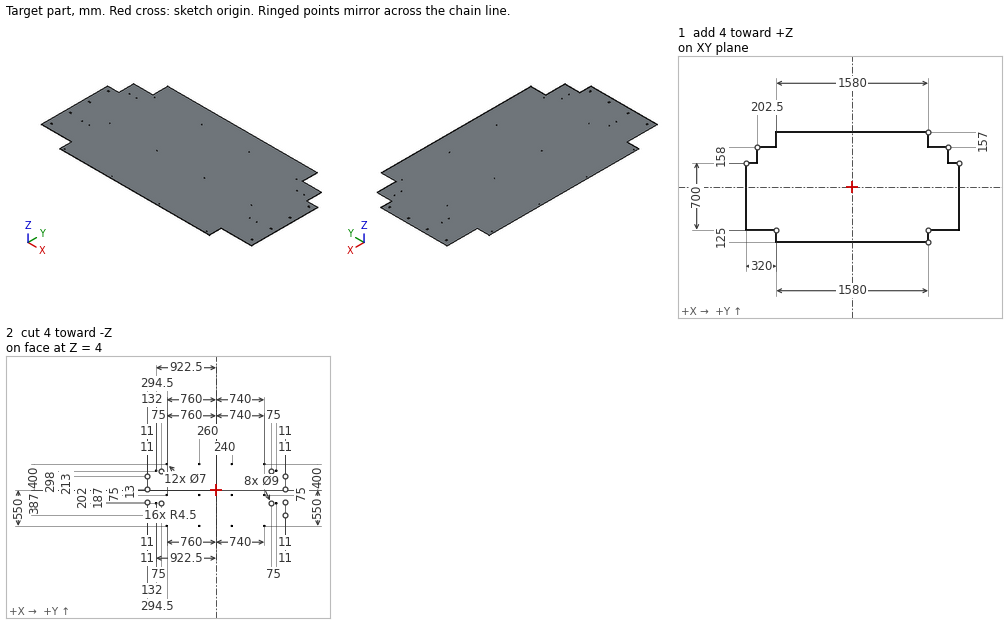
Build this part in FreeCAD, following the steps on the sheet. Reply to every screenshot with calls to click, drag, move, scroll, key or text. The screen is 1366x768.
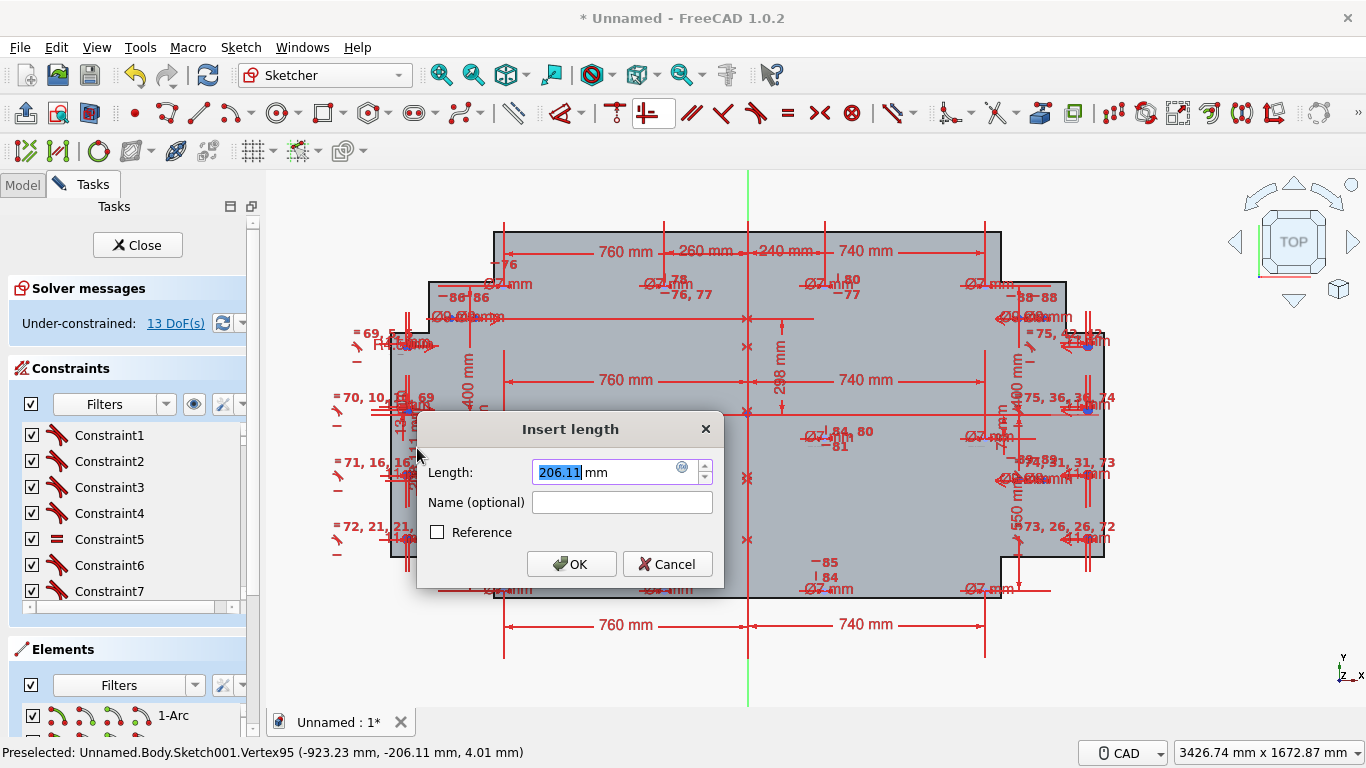
text(202)
key(Return)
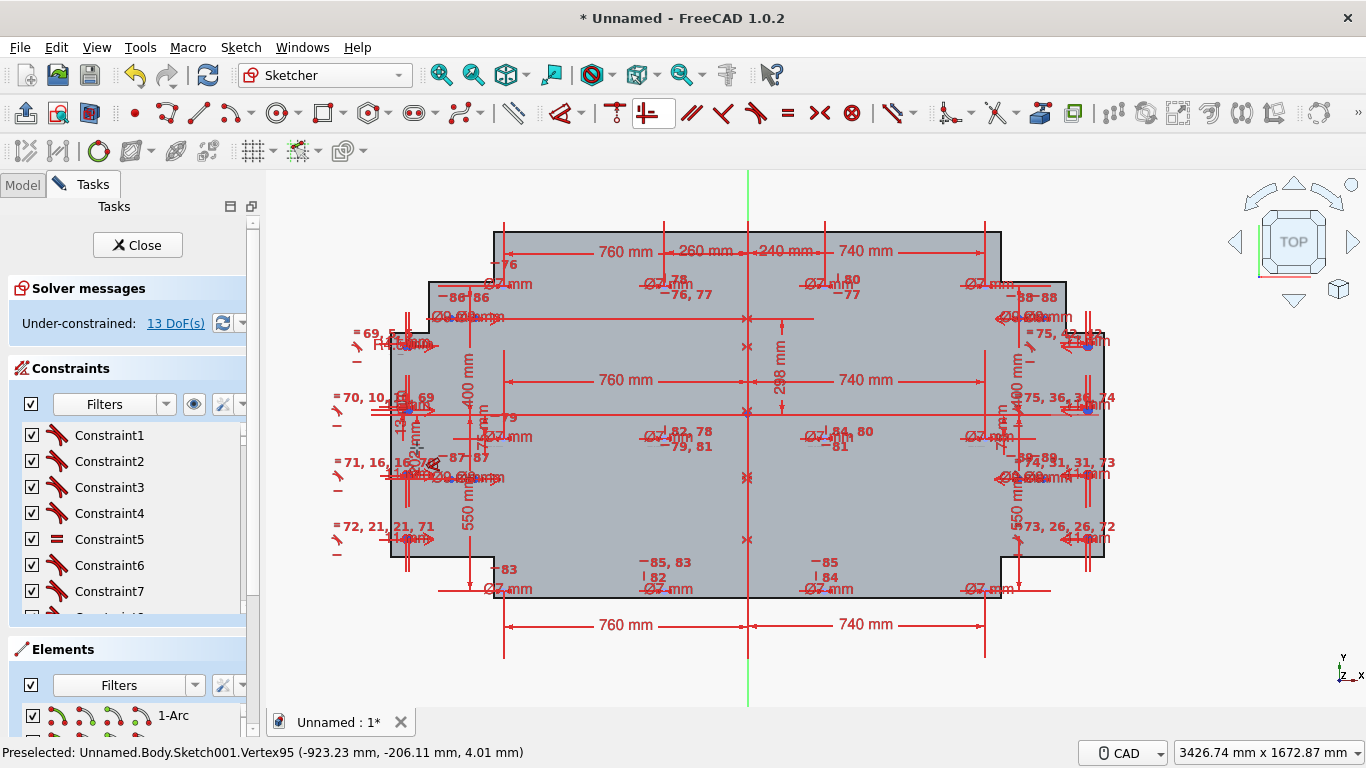
scroll(451, 319, up, 3)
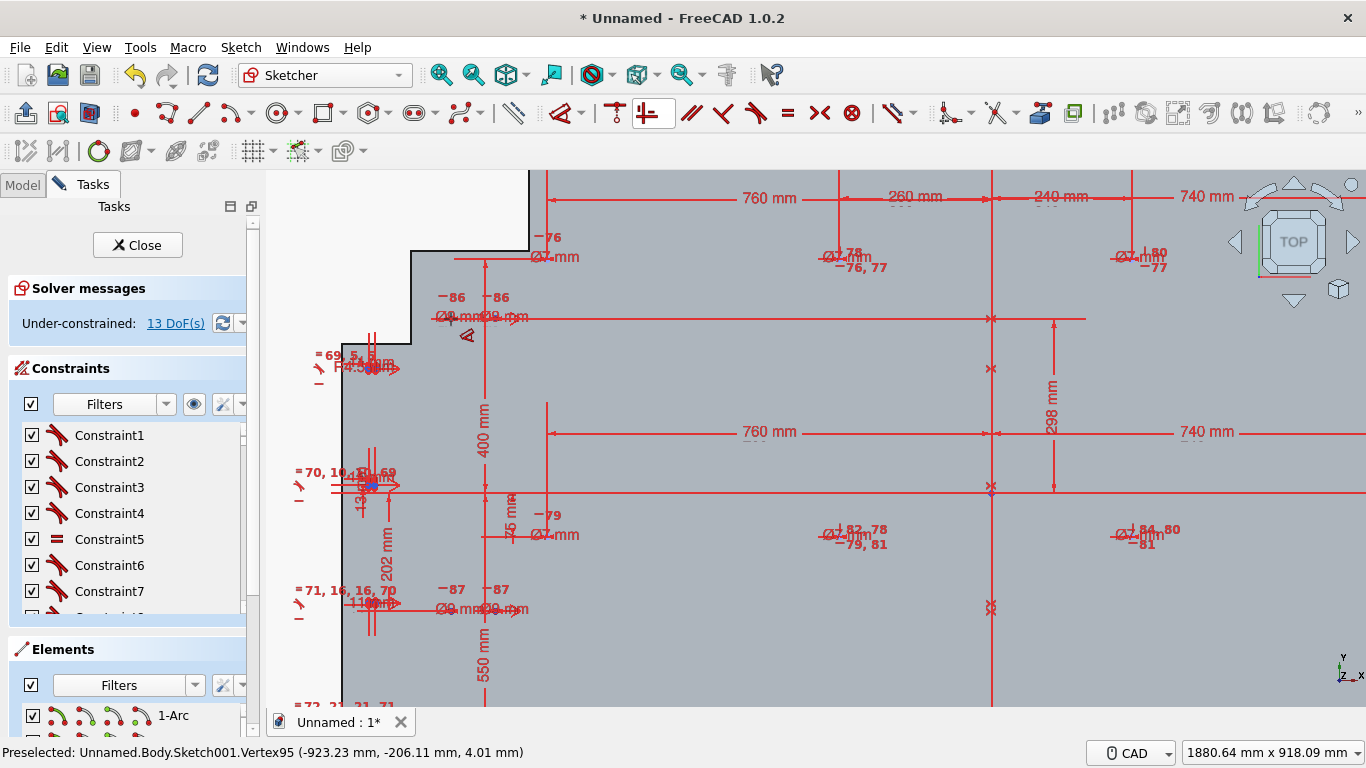
click(452, 319)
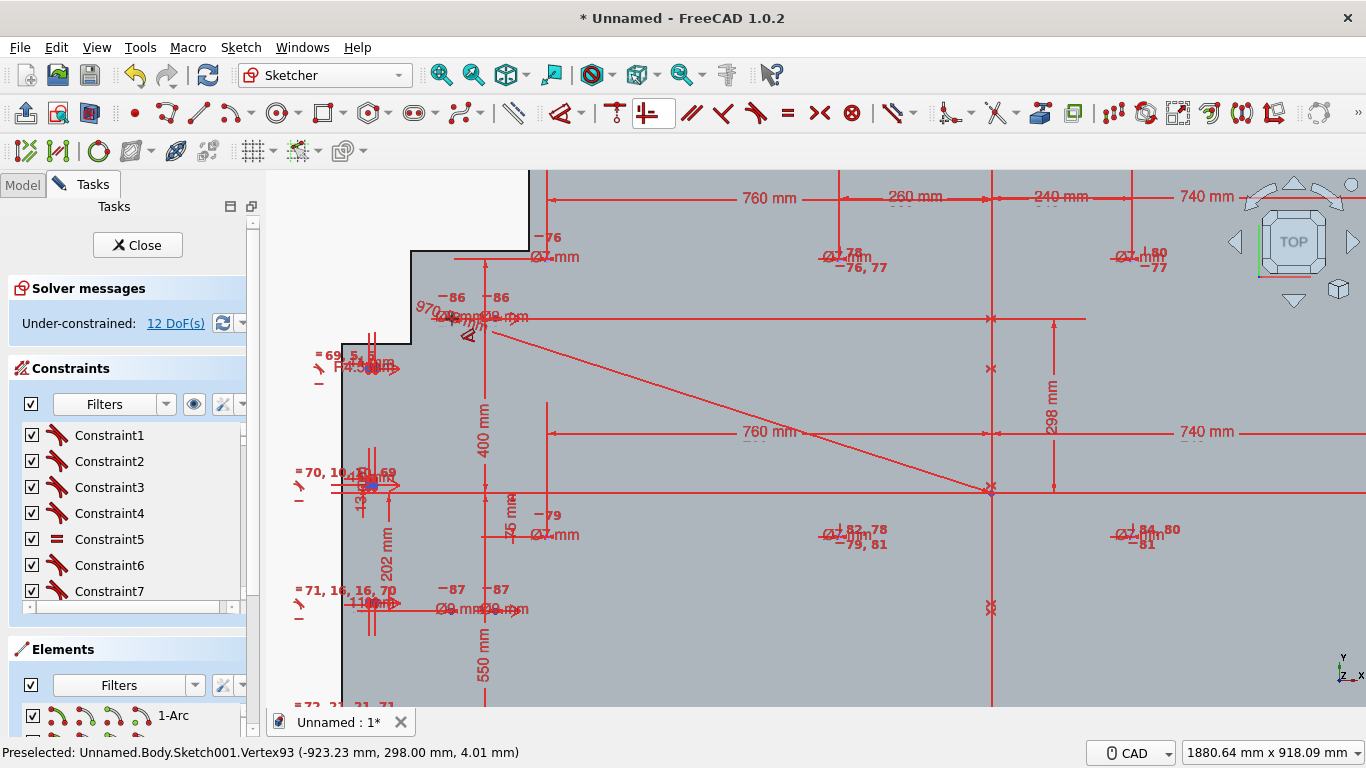
click(496, 319)
click(474, 285)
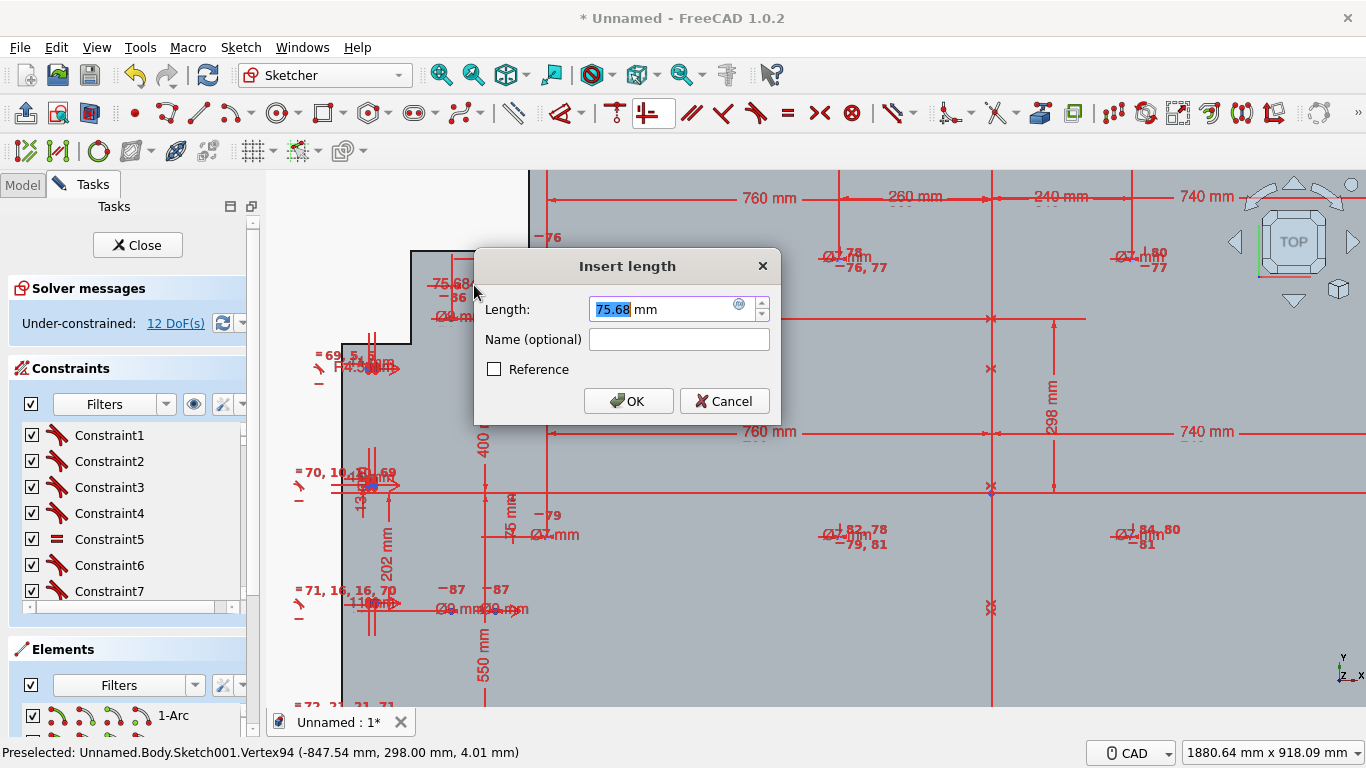
text(75)
key(Return)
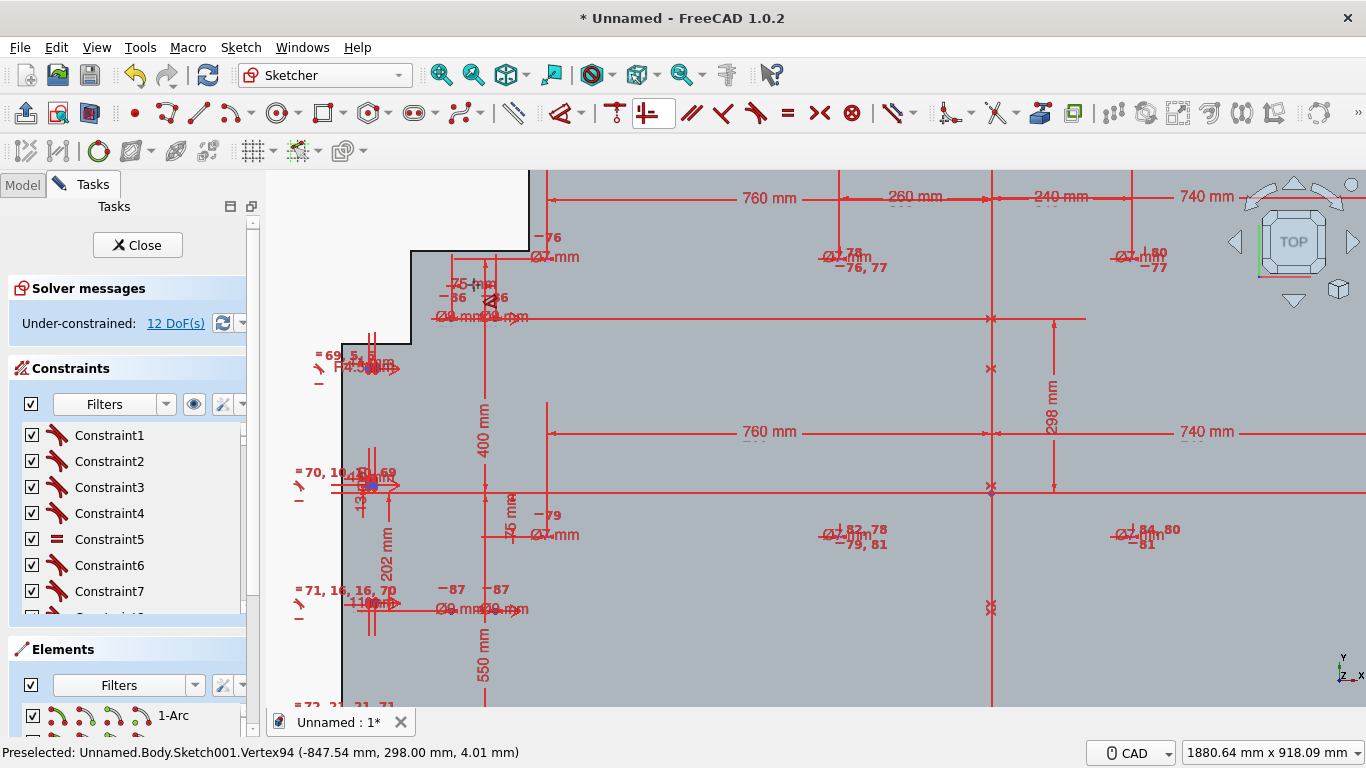
click(452, 611)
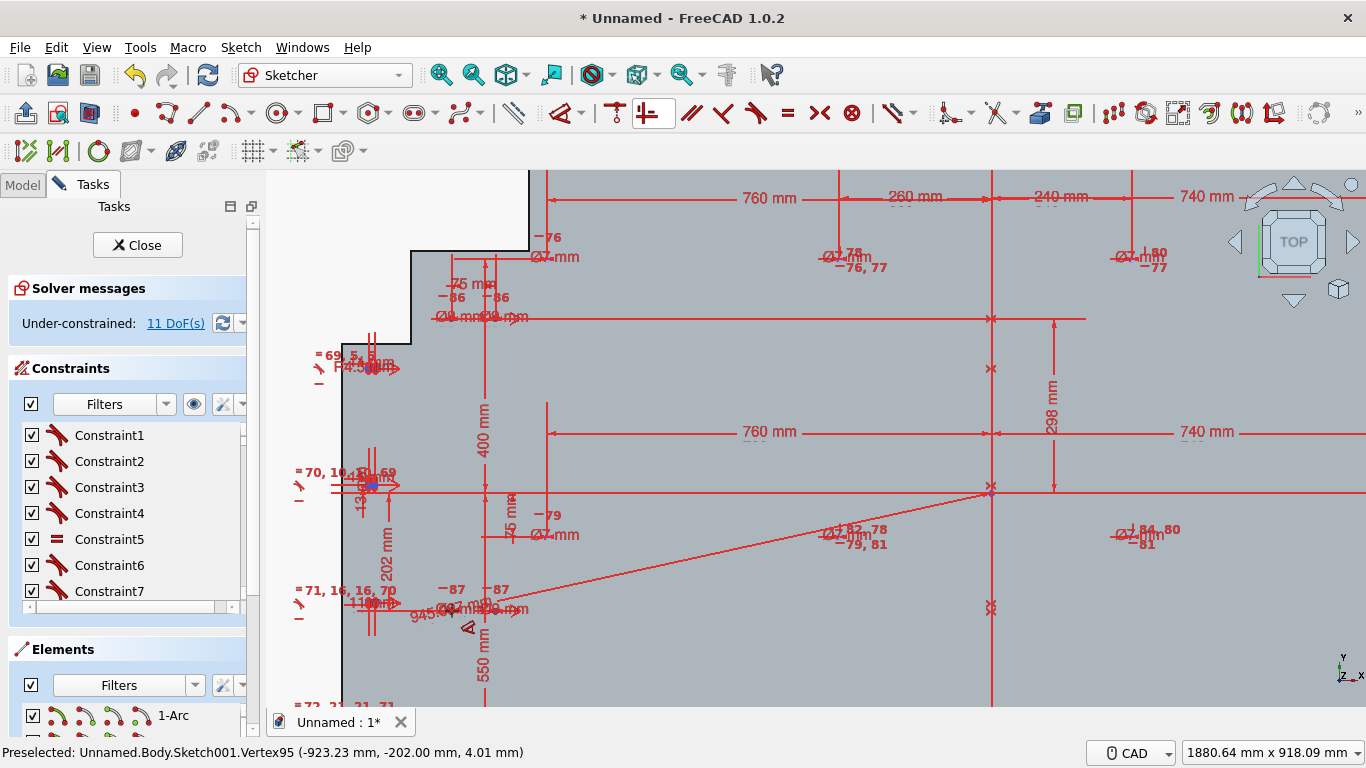
click(496, 611)
click(474, 577)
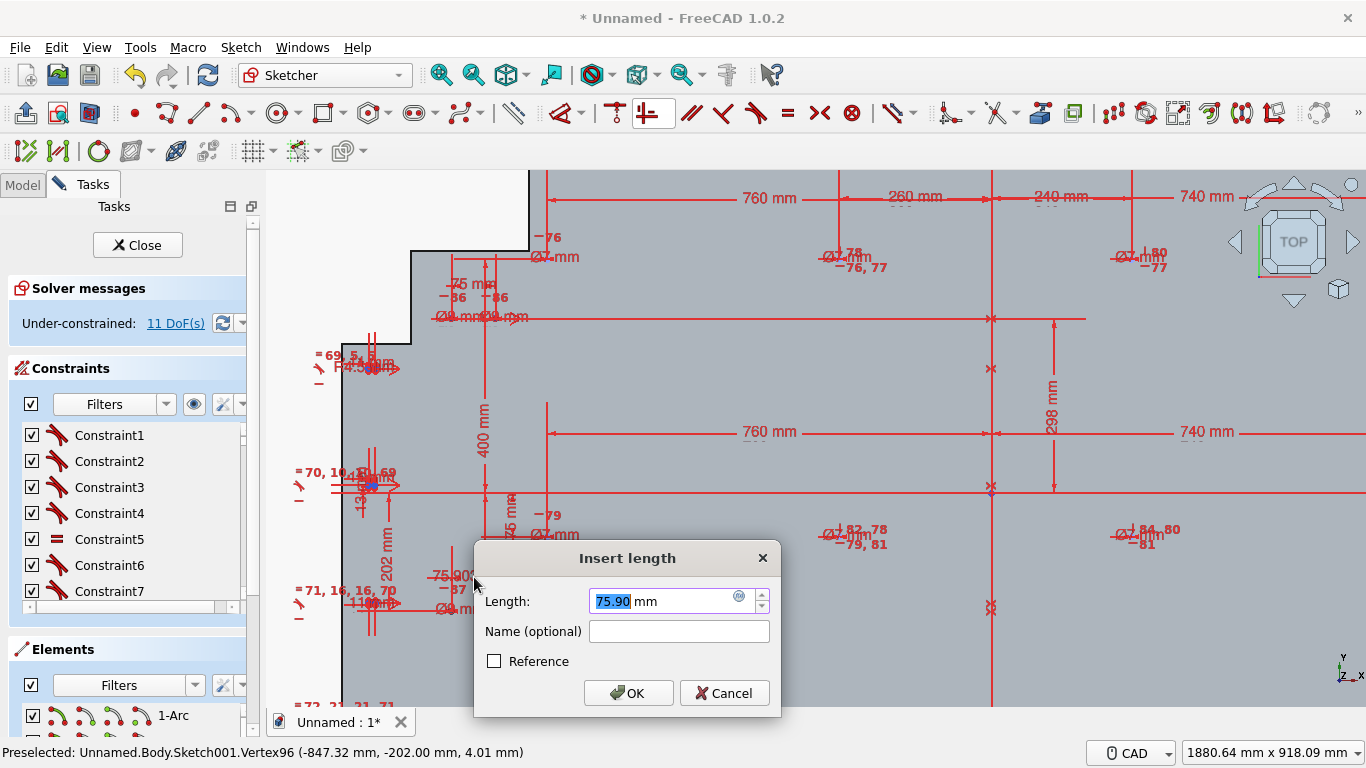
text(75)
key(Return)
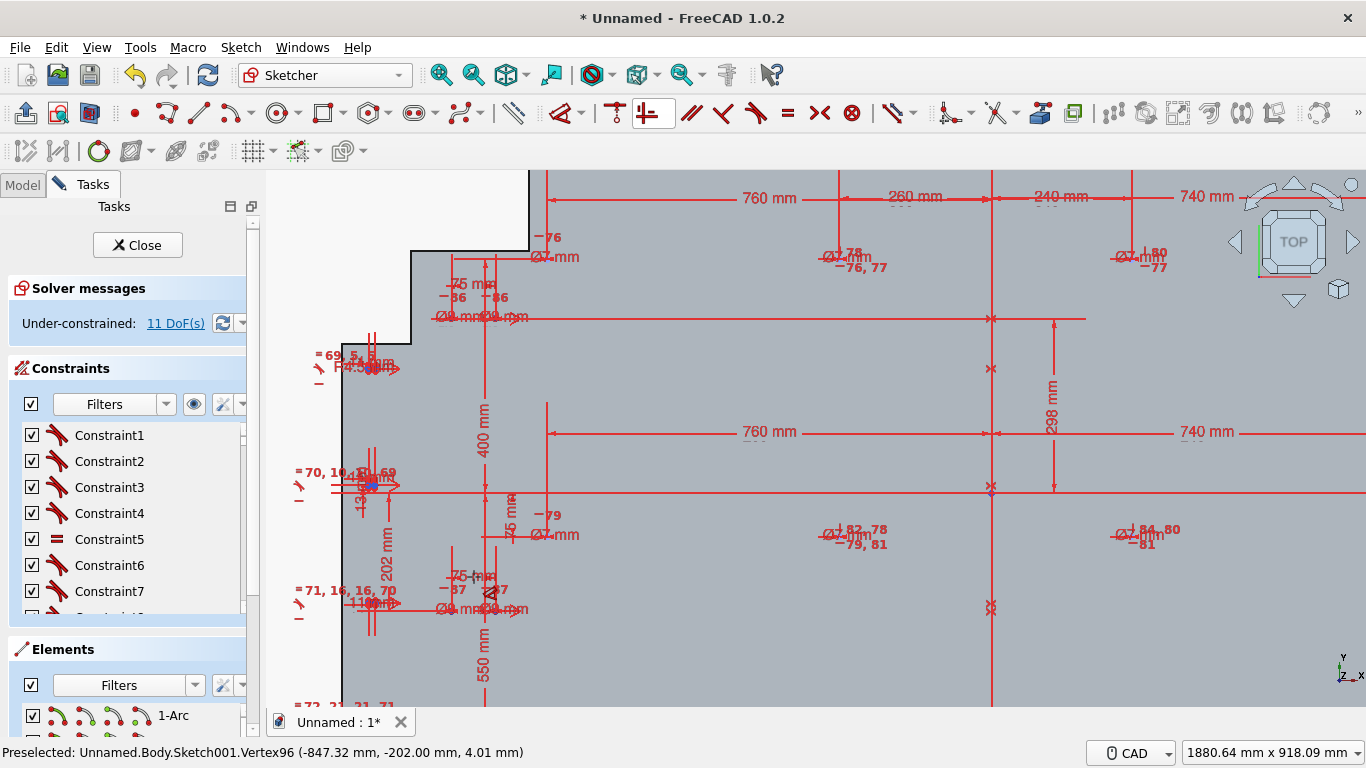
scroll(451, 319, down, 3)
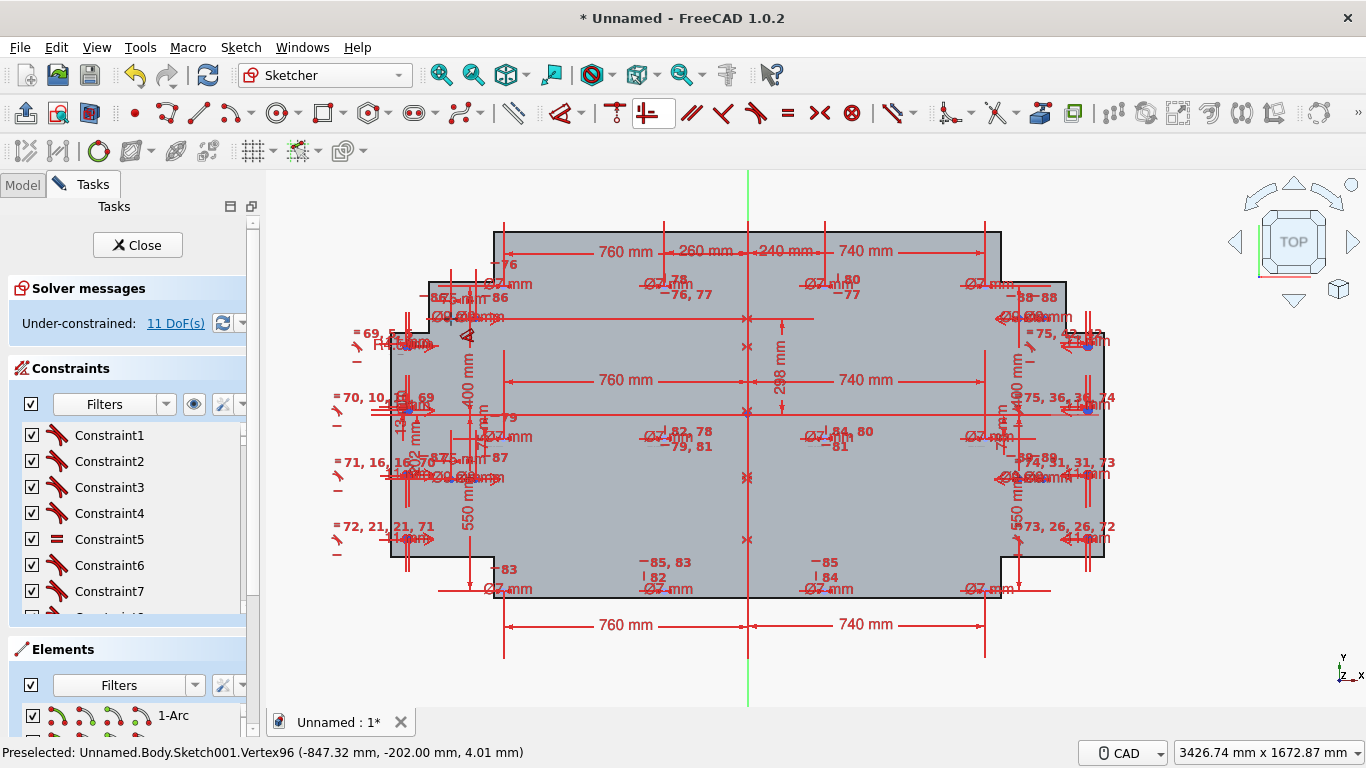
scroll(1020, 319, up, 3)